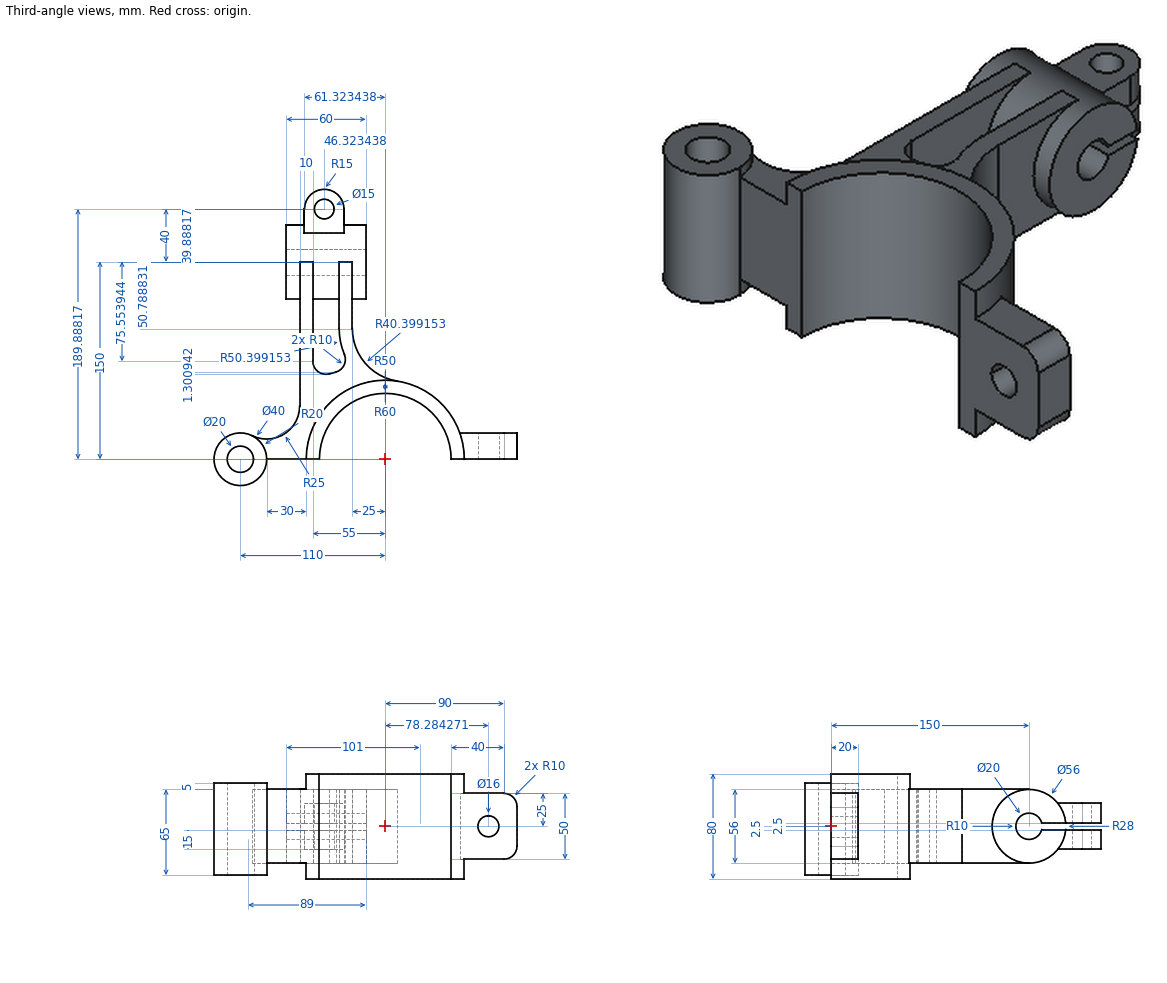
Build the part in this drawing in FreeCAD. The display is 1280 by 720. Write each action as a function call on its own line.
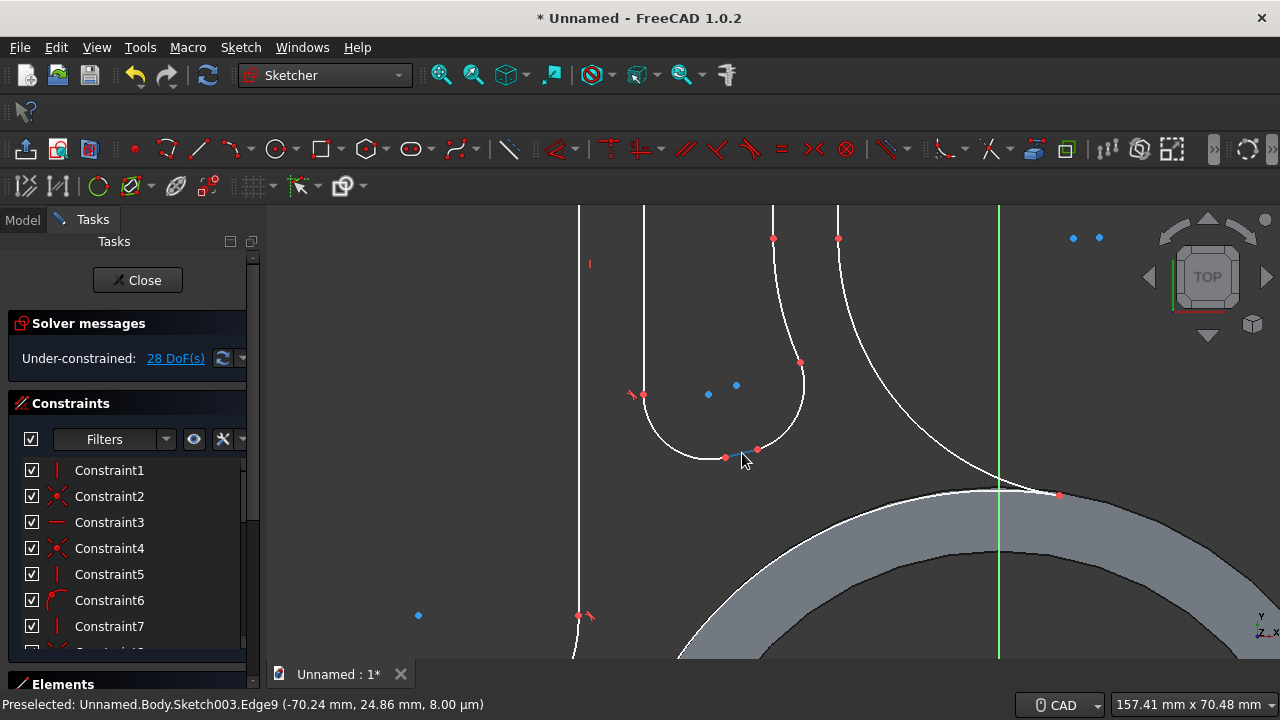
click(741, 453)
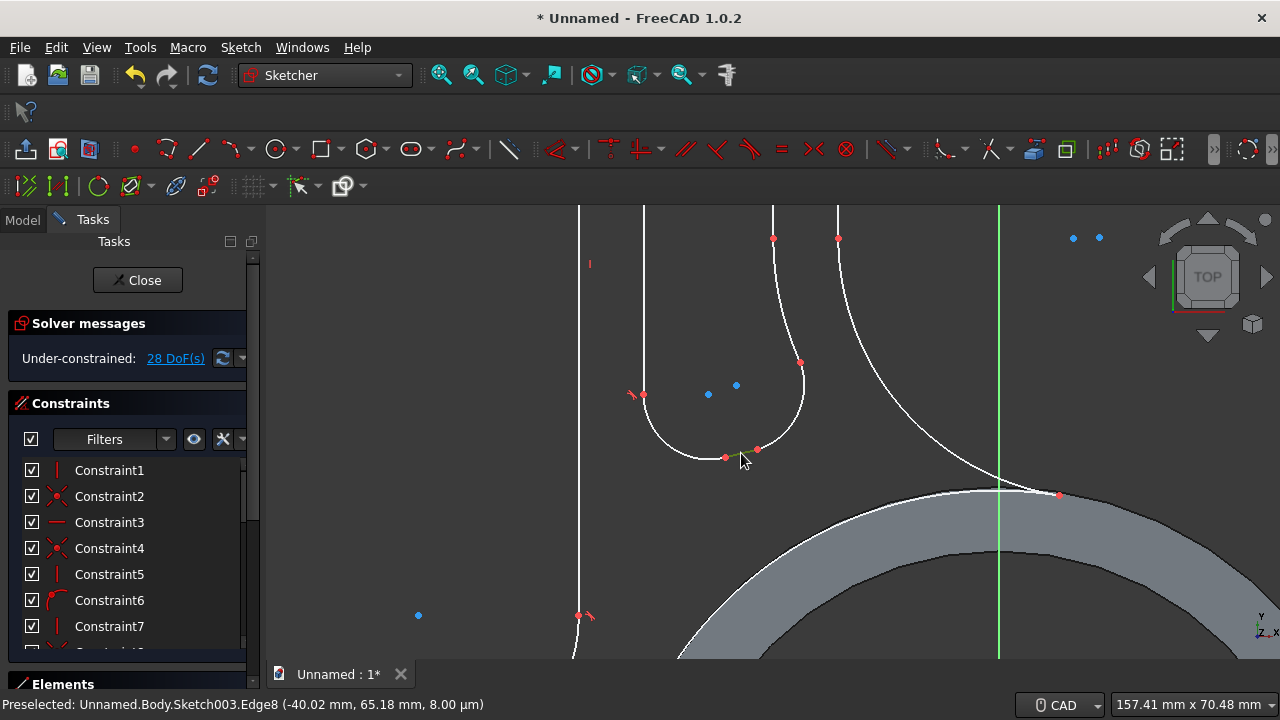
click(785, 433)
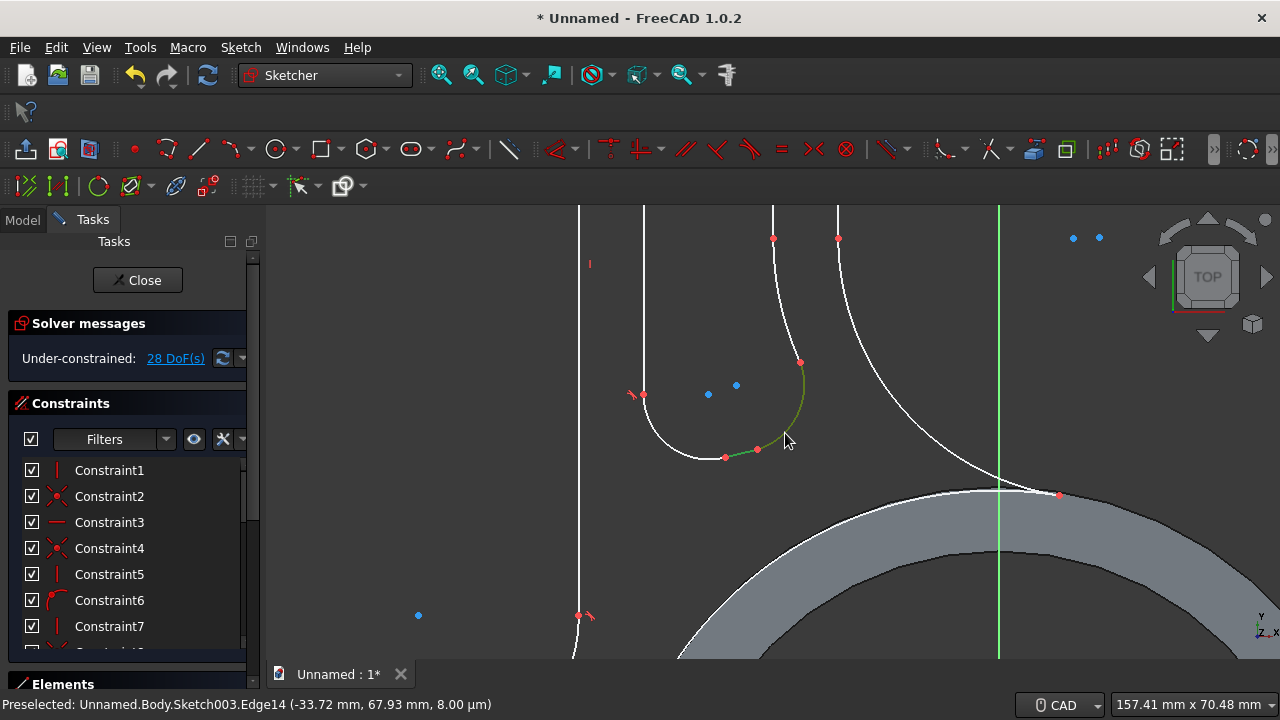
click(750, 150)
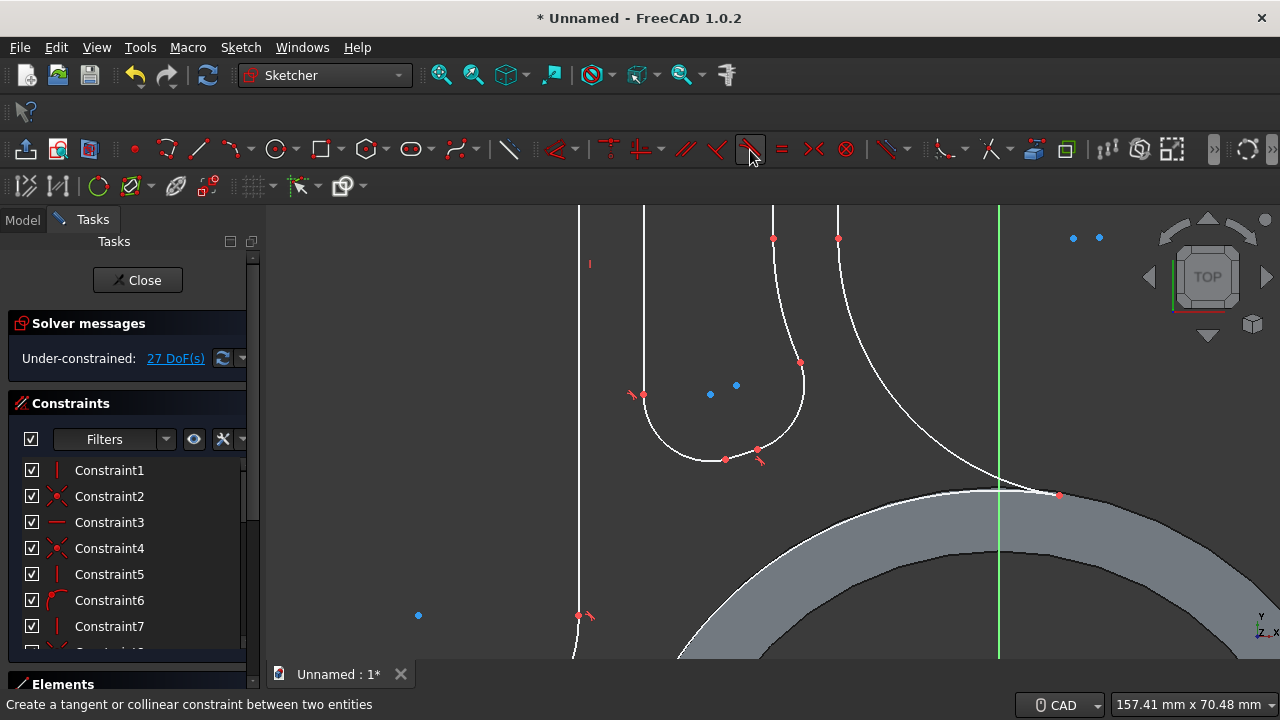
scroll(748, 453, up, 2)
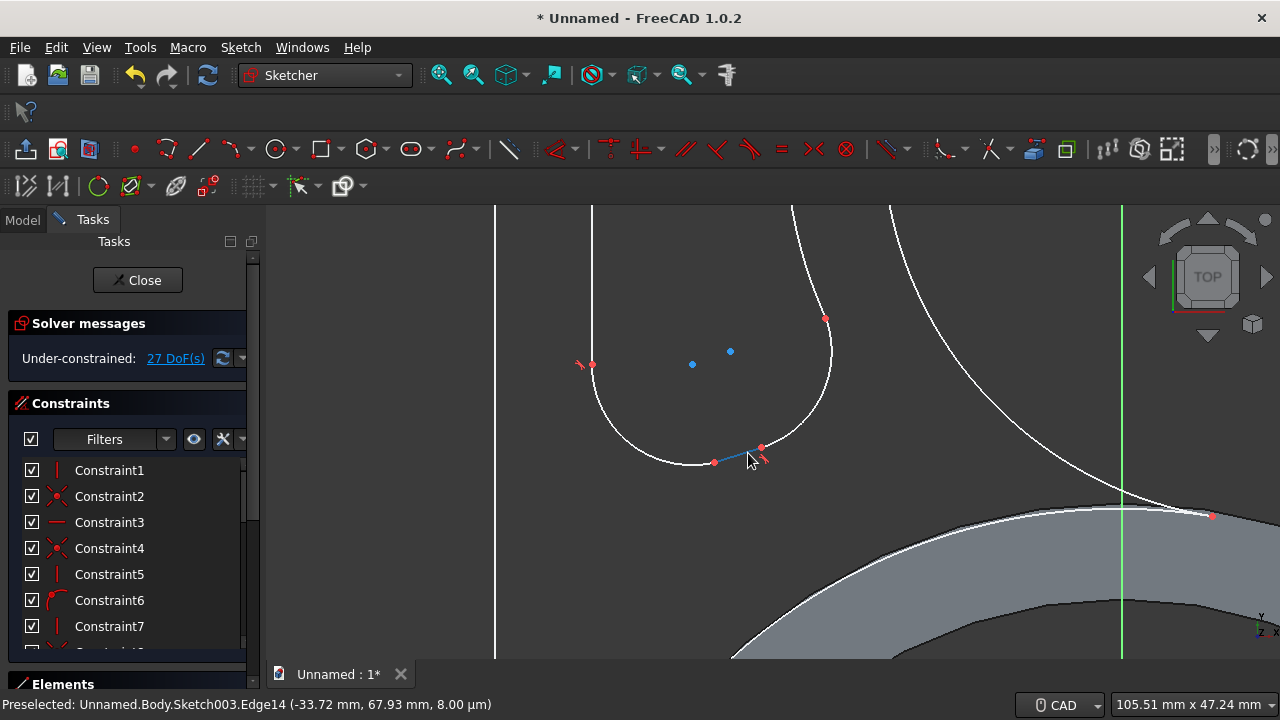
click(747, 452)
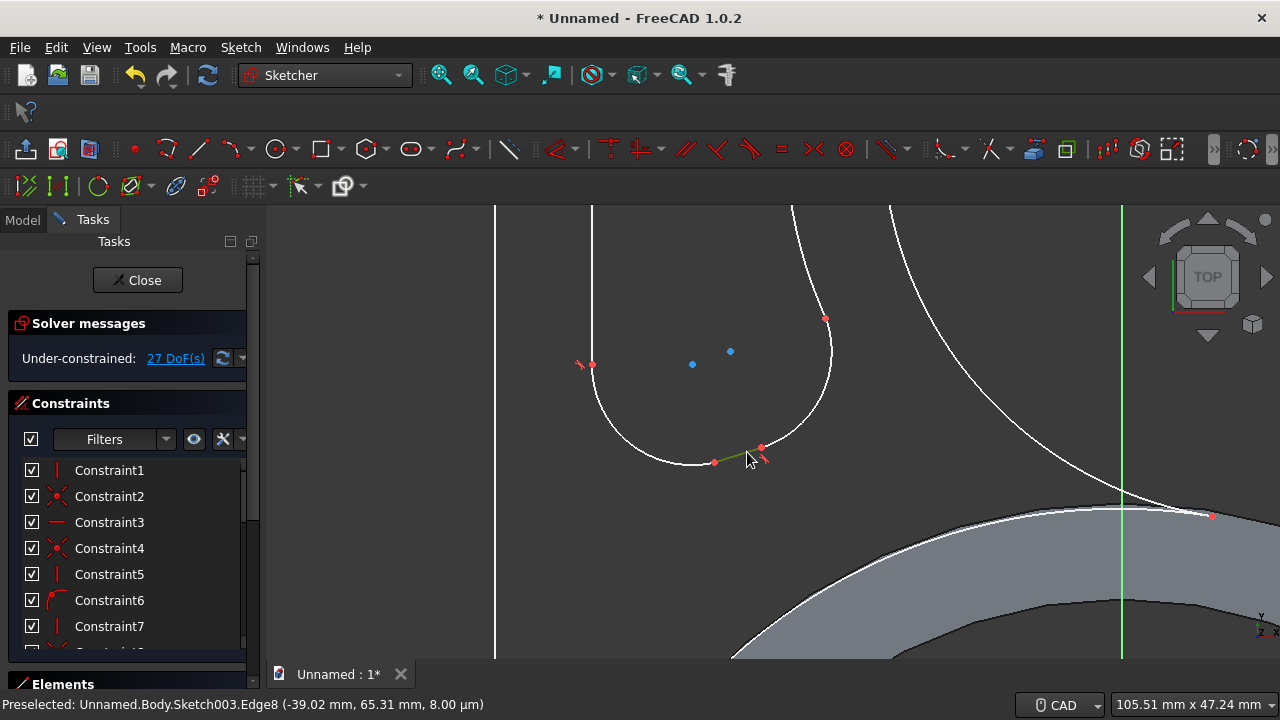
scroll(711, 450, down, 8)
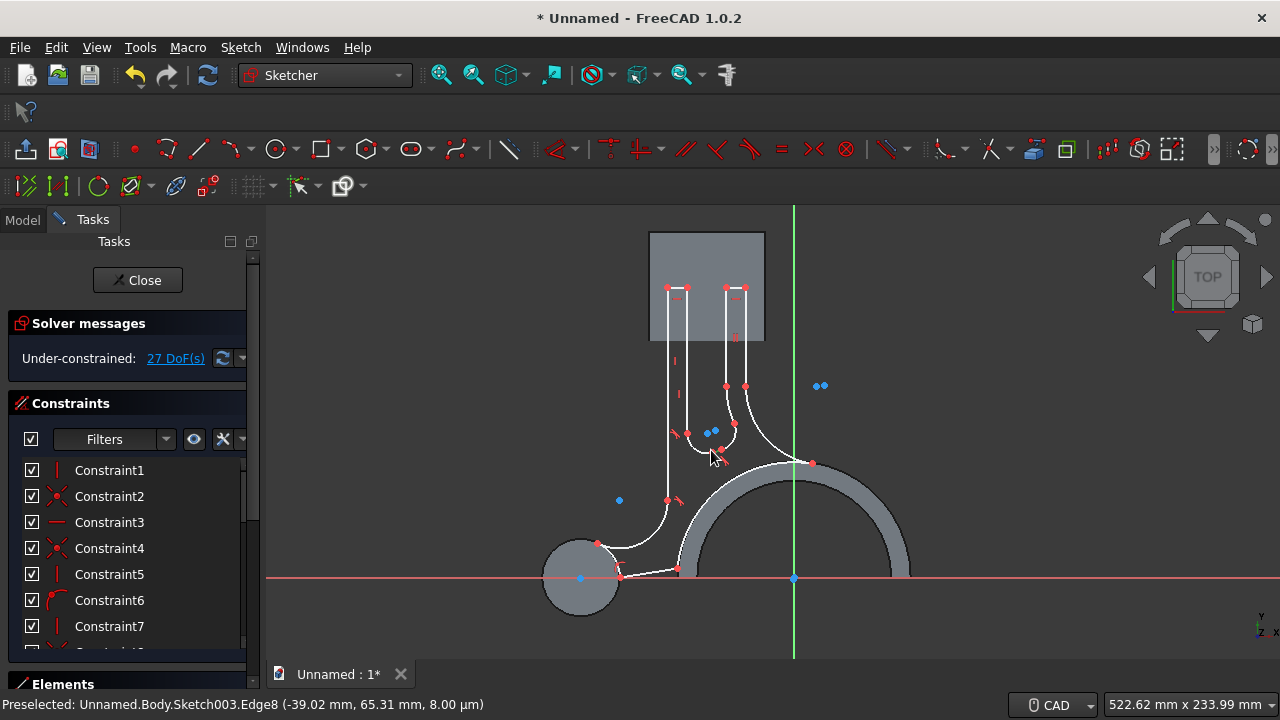
scroll(690, 444, up, 2)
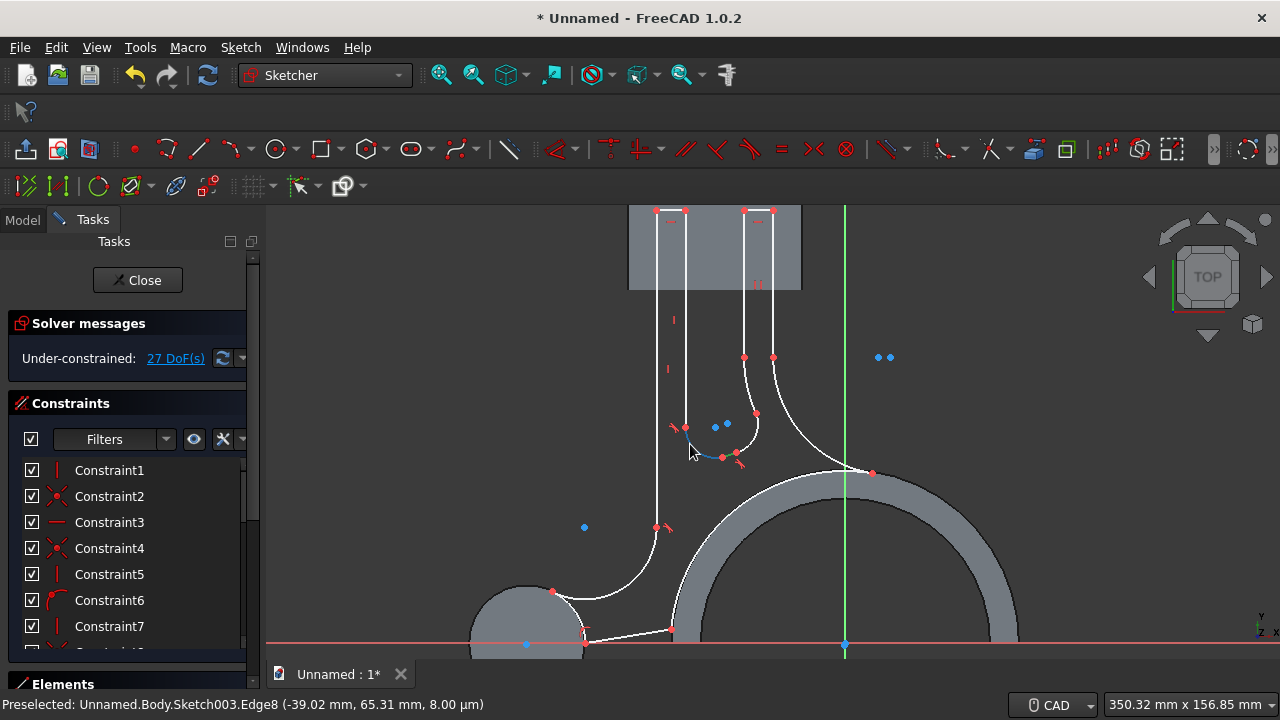
click(690, 443)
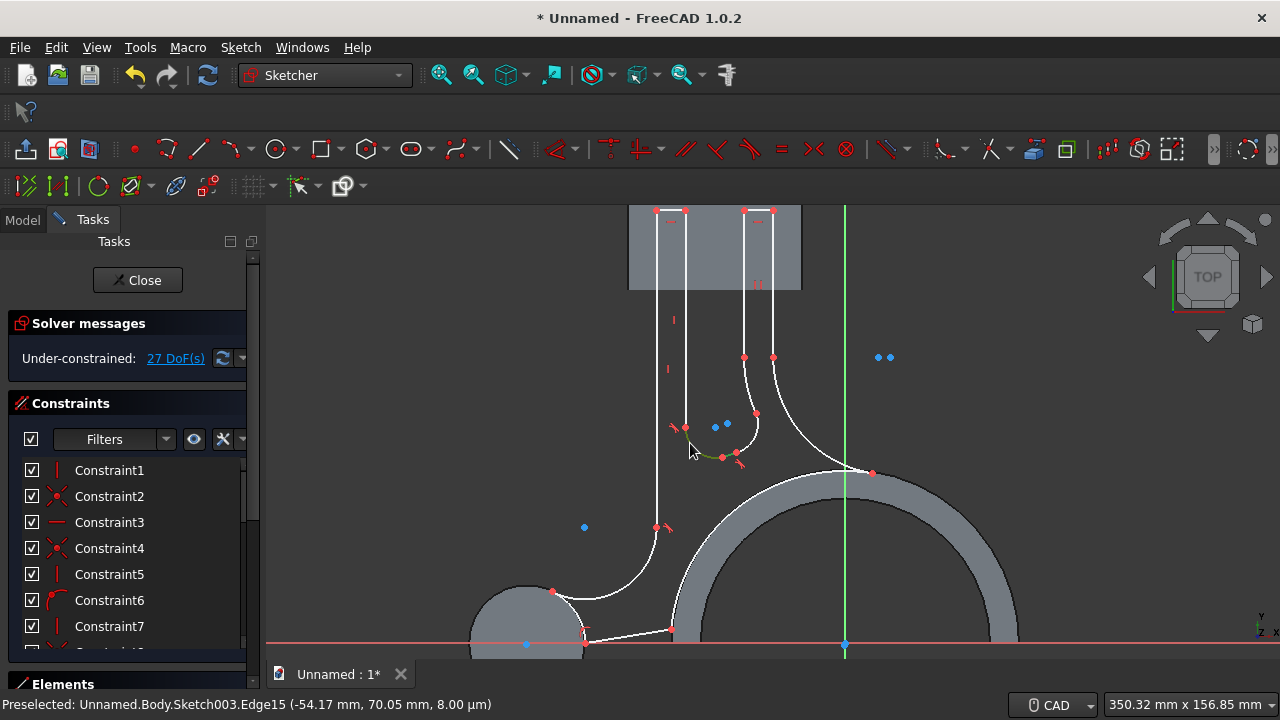
key(t)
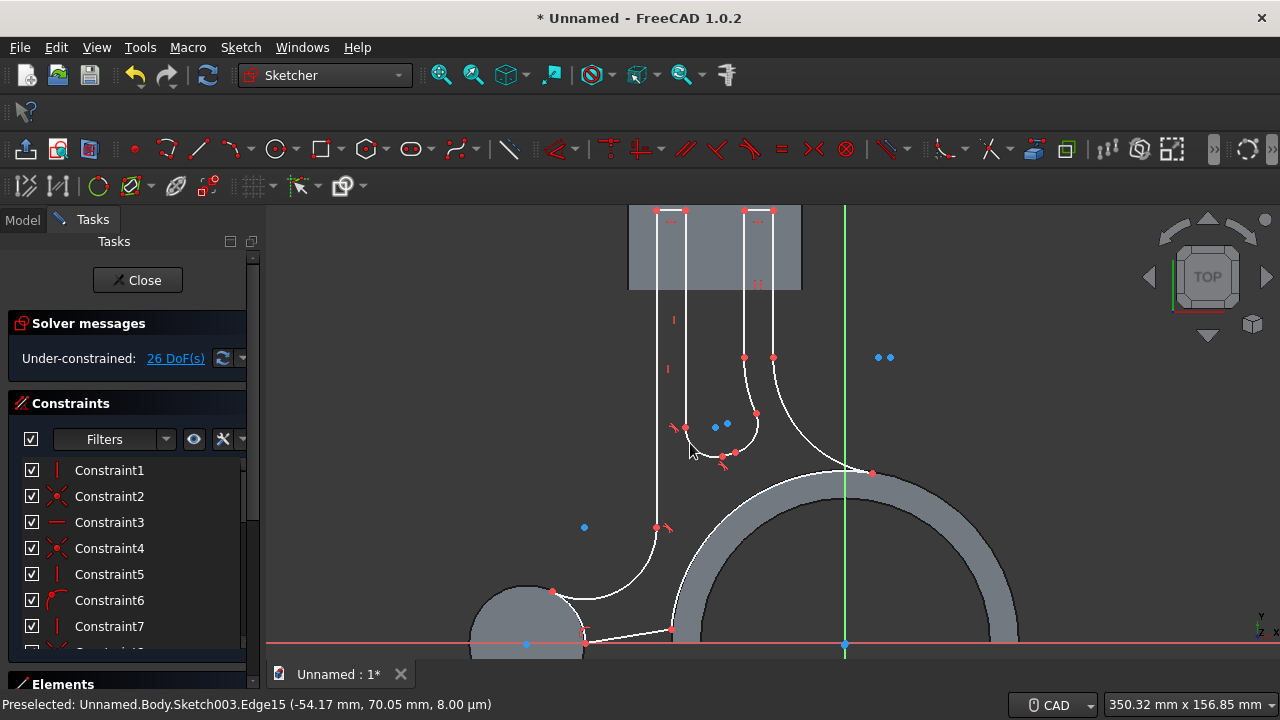
click(595, 599)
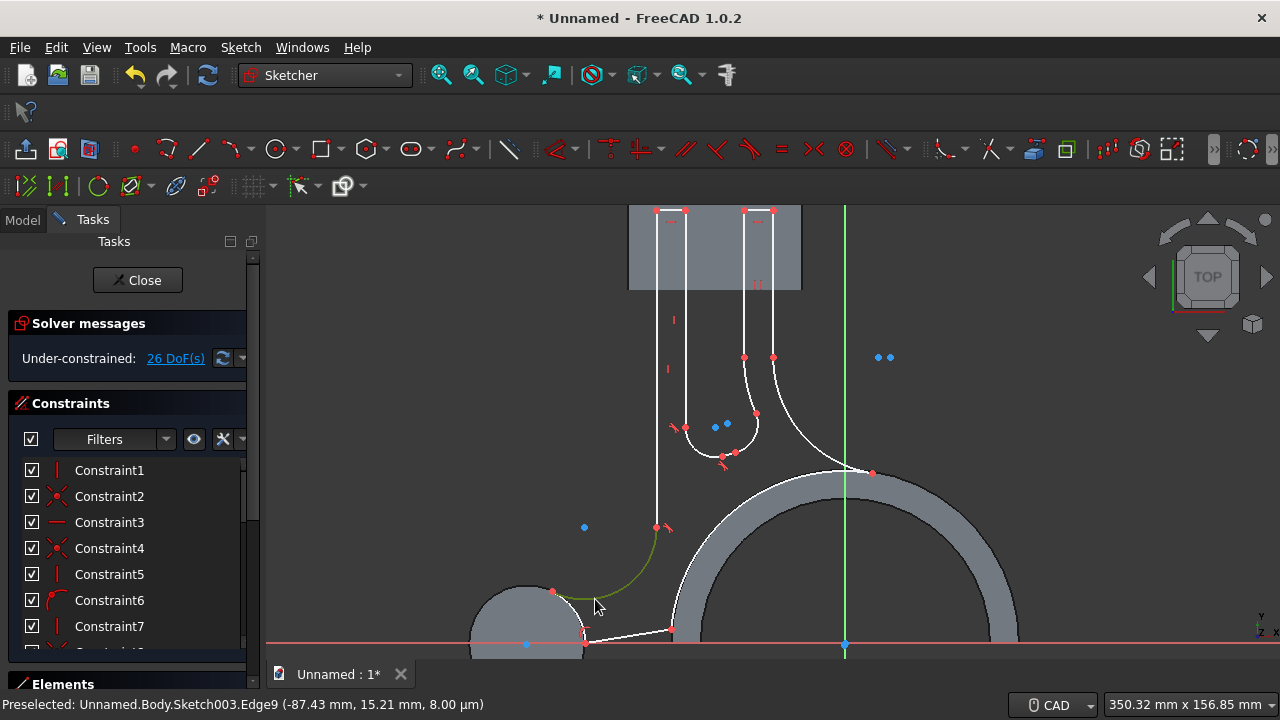
click(582, 624)